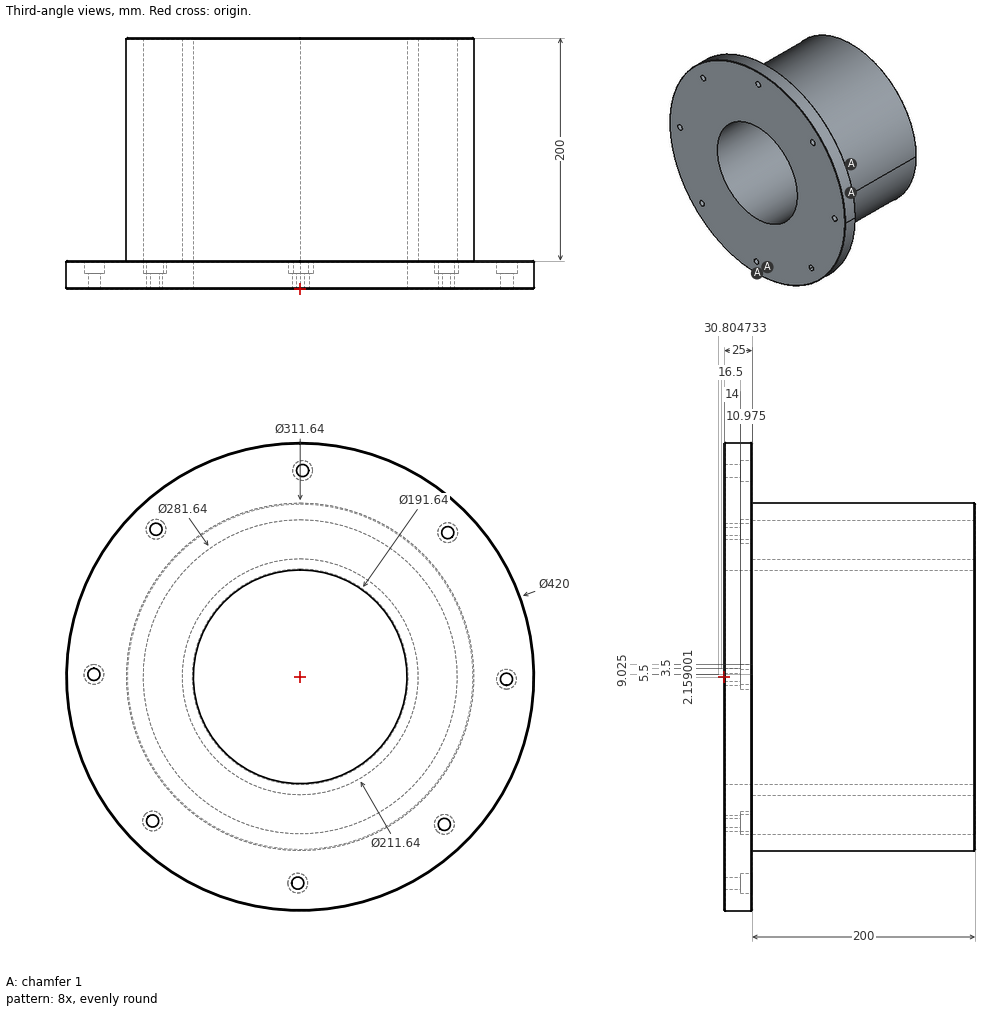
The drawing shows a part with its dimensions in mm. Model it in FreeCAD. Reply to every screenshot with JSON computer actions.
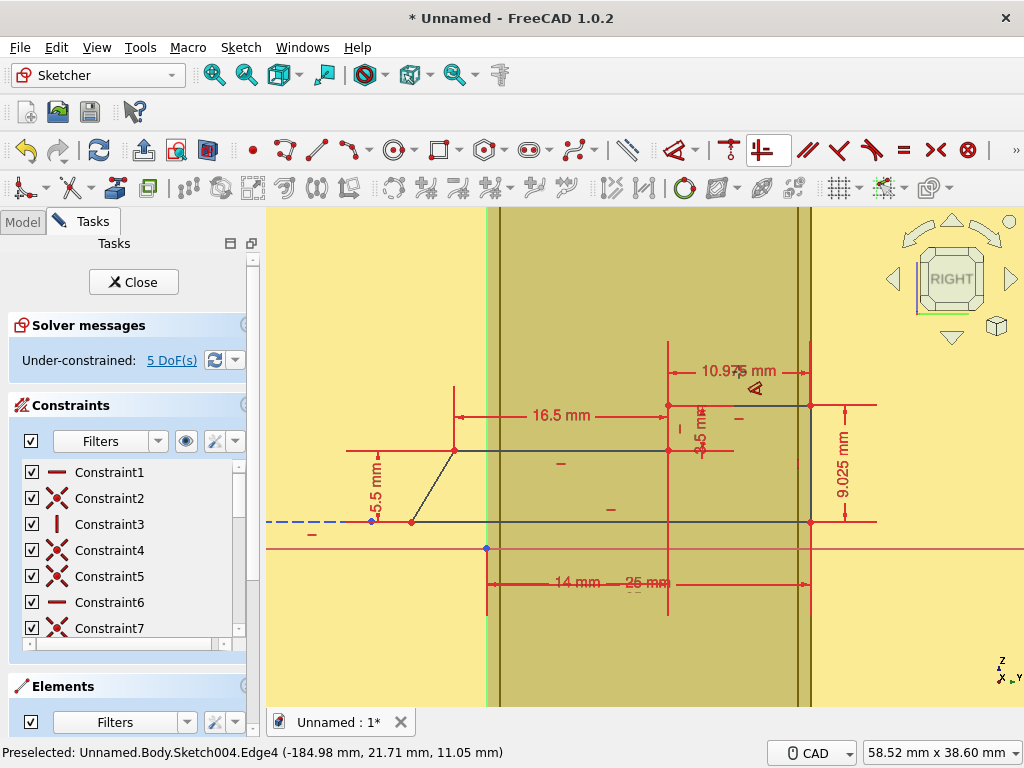
{"action": "left_click", "coordinate": [531, 522]}
{"action": "left_click", "coordinate": [611, 488]}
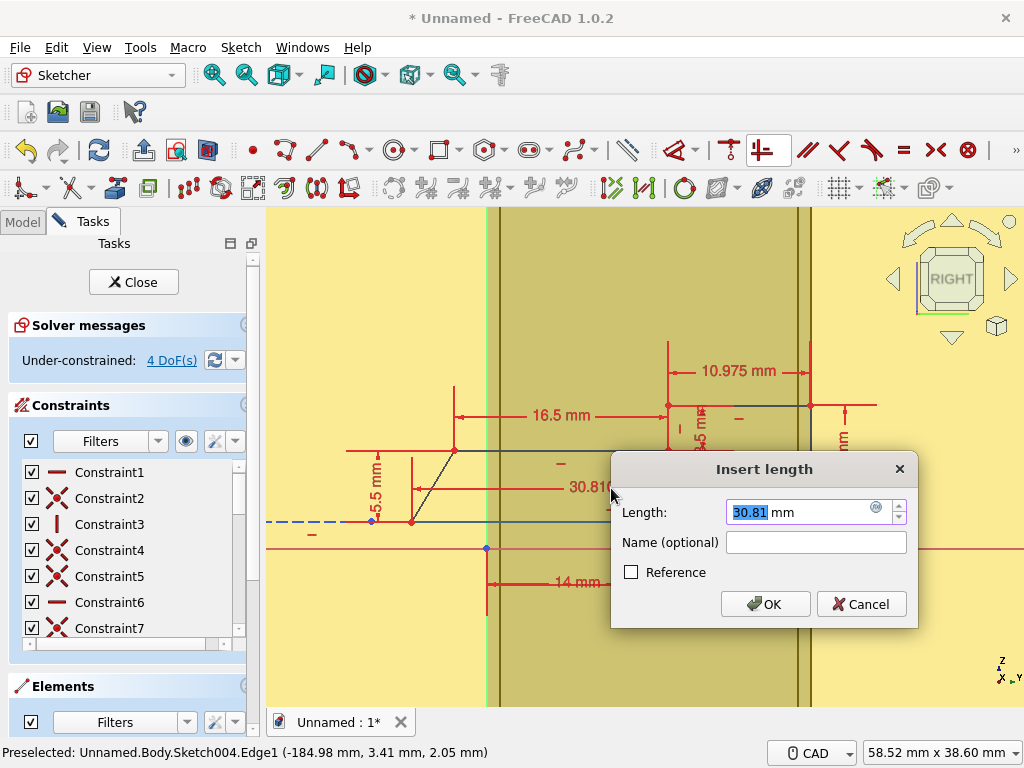
{"action": "type", "text": "30.804733"}
{"action": "key", "text": "Return"}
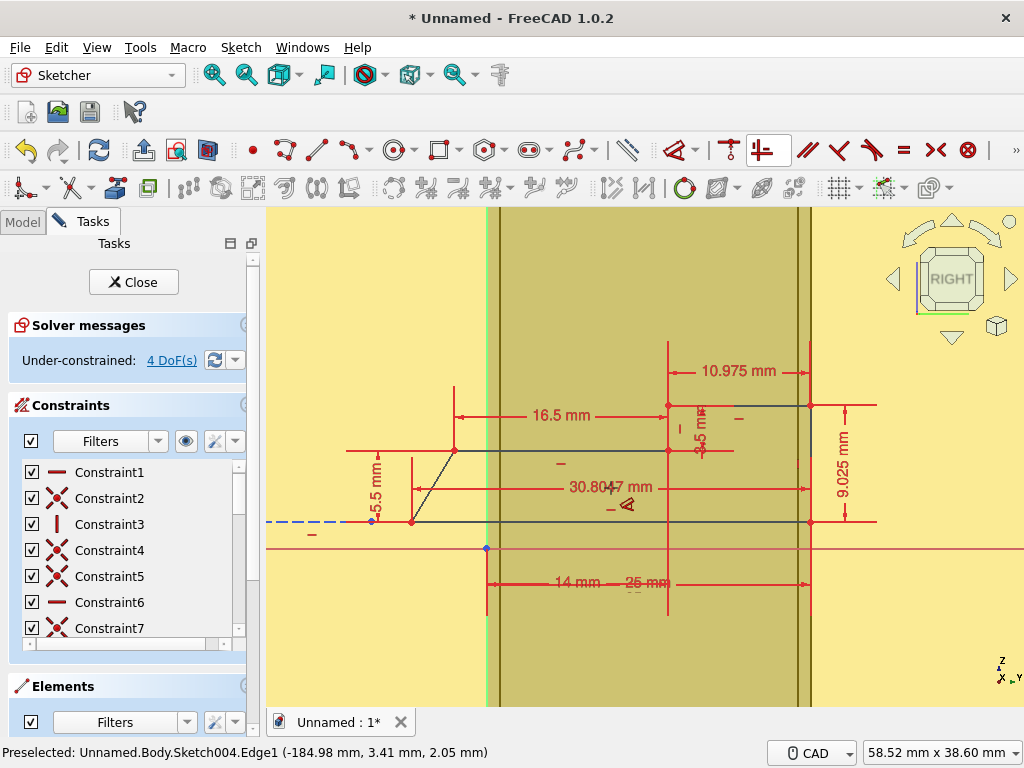
{"action": "scroll", "coordinate": [412, 522], "scroll_direction": "up", "scroll_amount": 2}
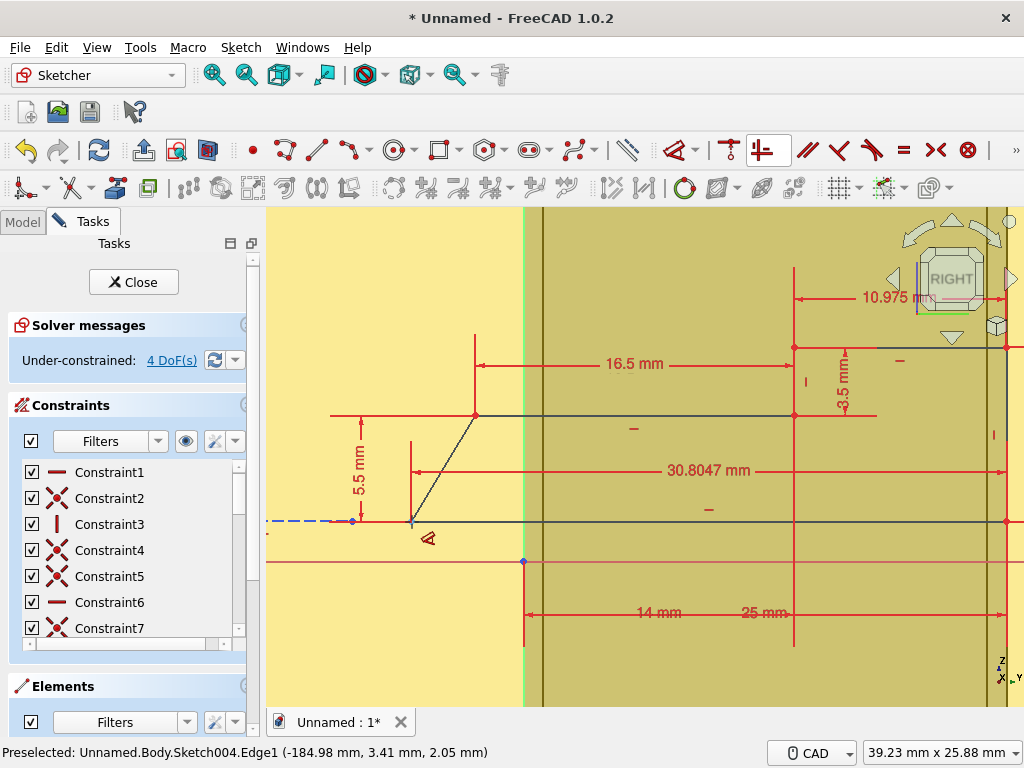
{"action": "left_click", "coordinate": [411, 522]}
{"action": "left_click", "coordinate": [377, 542]}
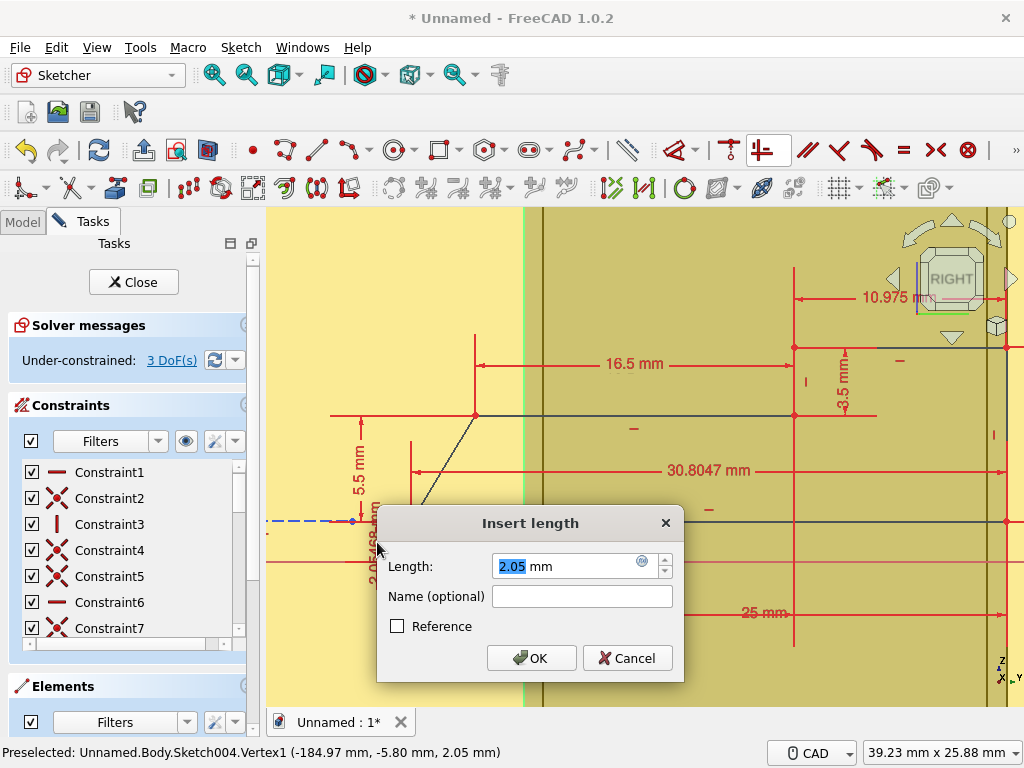
{"action": "type", "text": "2.159001"}
{"action": "key", "text": "Return"}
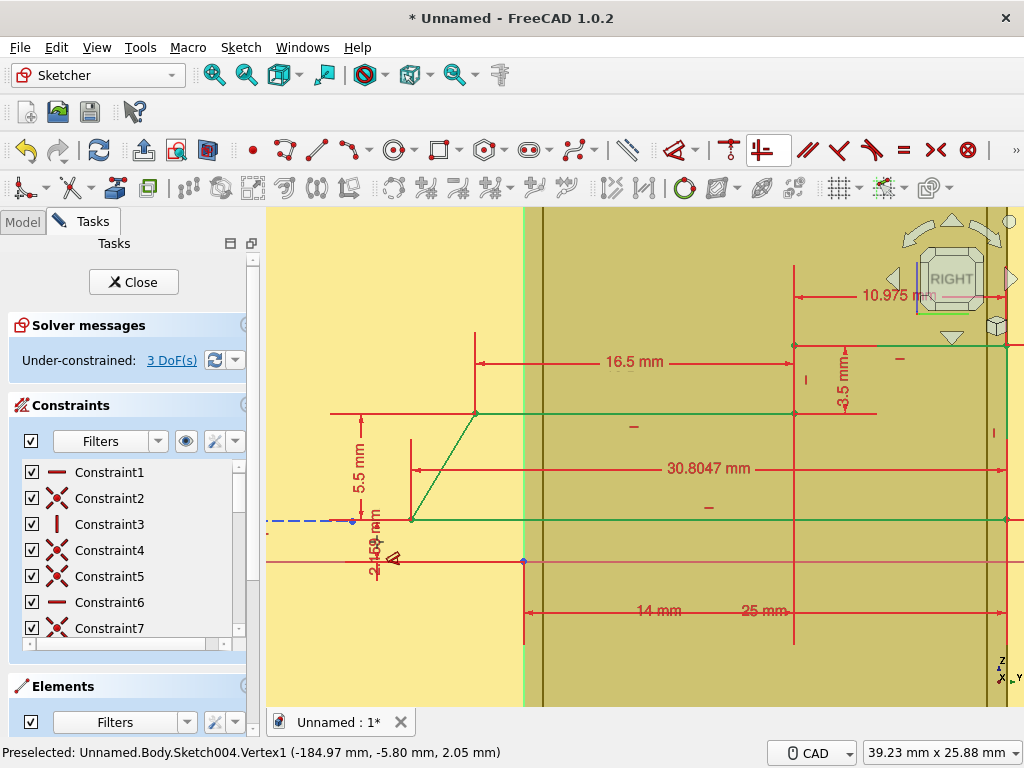
{"action": "left_click", "coordinate": [352, 521]}
{"action": "left_click", "coordinate": [558, 541]}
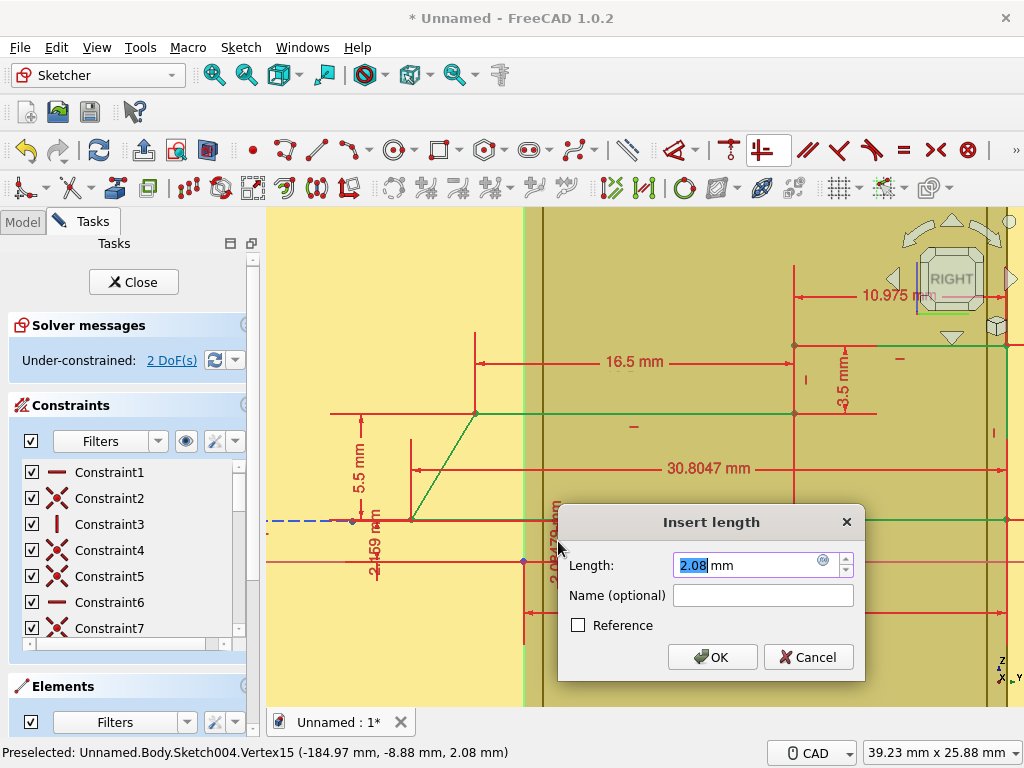
{"action": "type", "text": "2.159001"}
{"action": "key", "text": "Return"}
{"action": "key", "text": "Escape"}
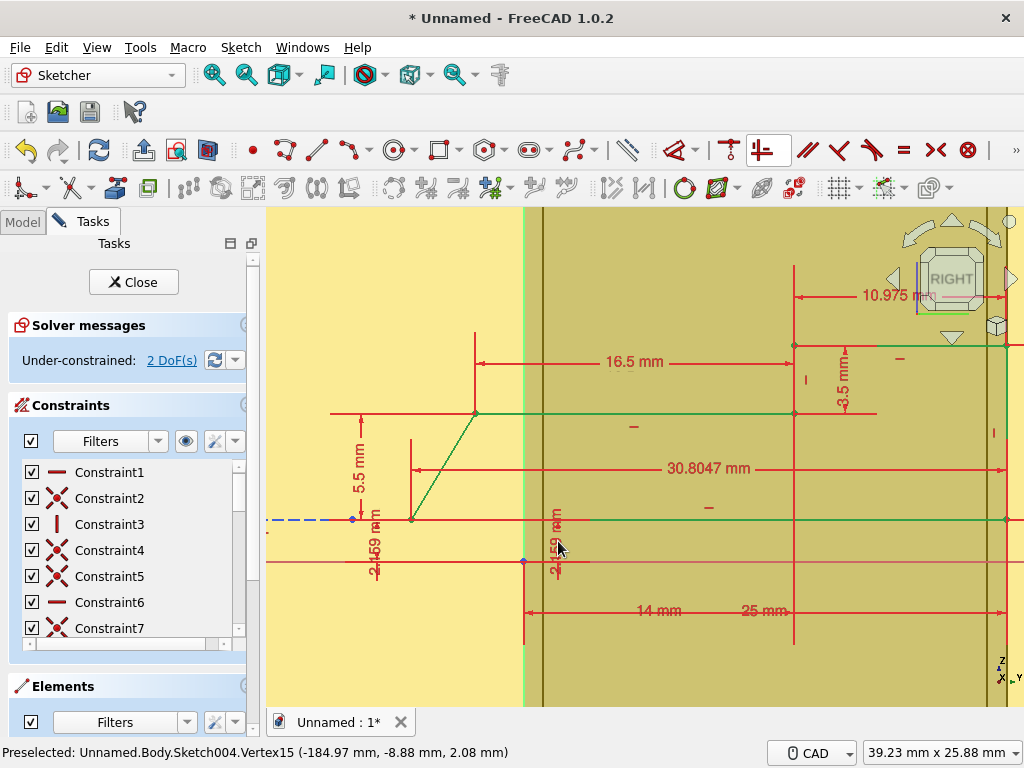
{"action": "left_click", "coordinate": [134, 282]}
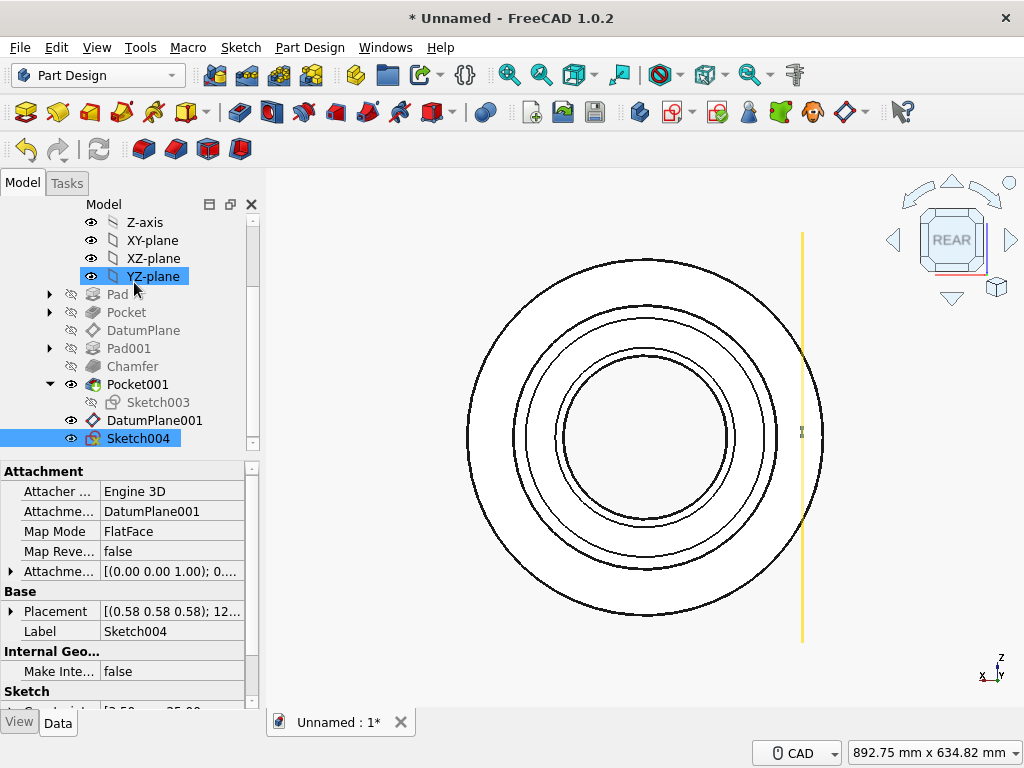
{"action": "left_click", "coordinate": [304, 112]}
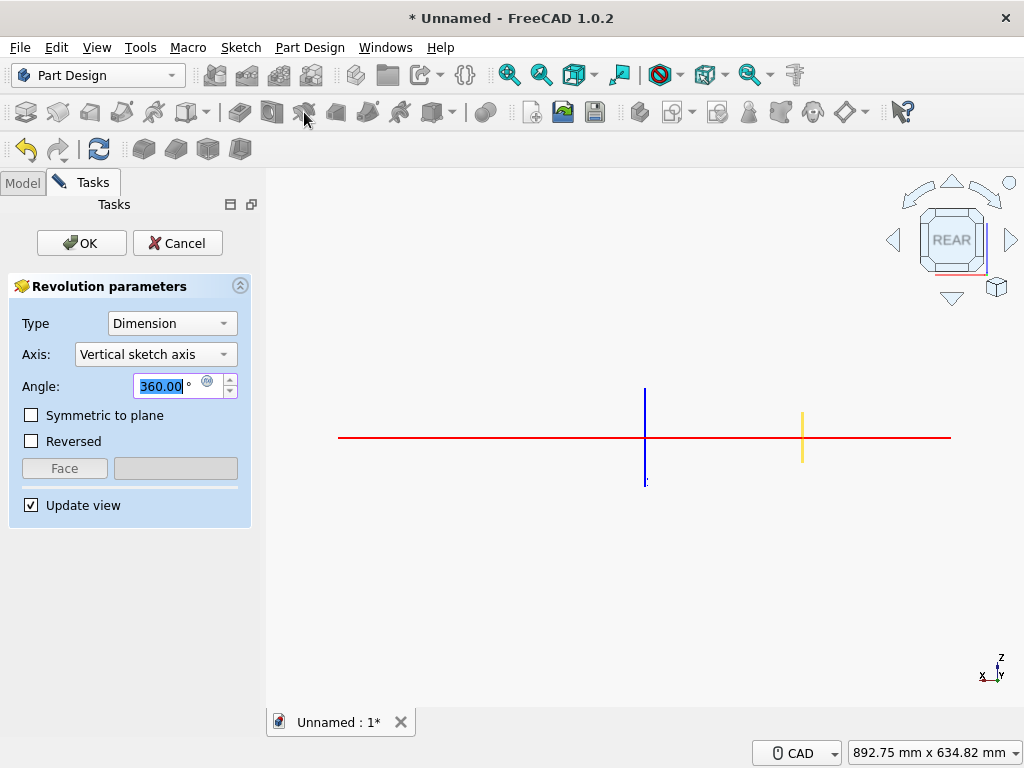
{"action": "left_click", "coordinate": [156, 354]}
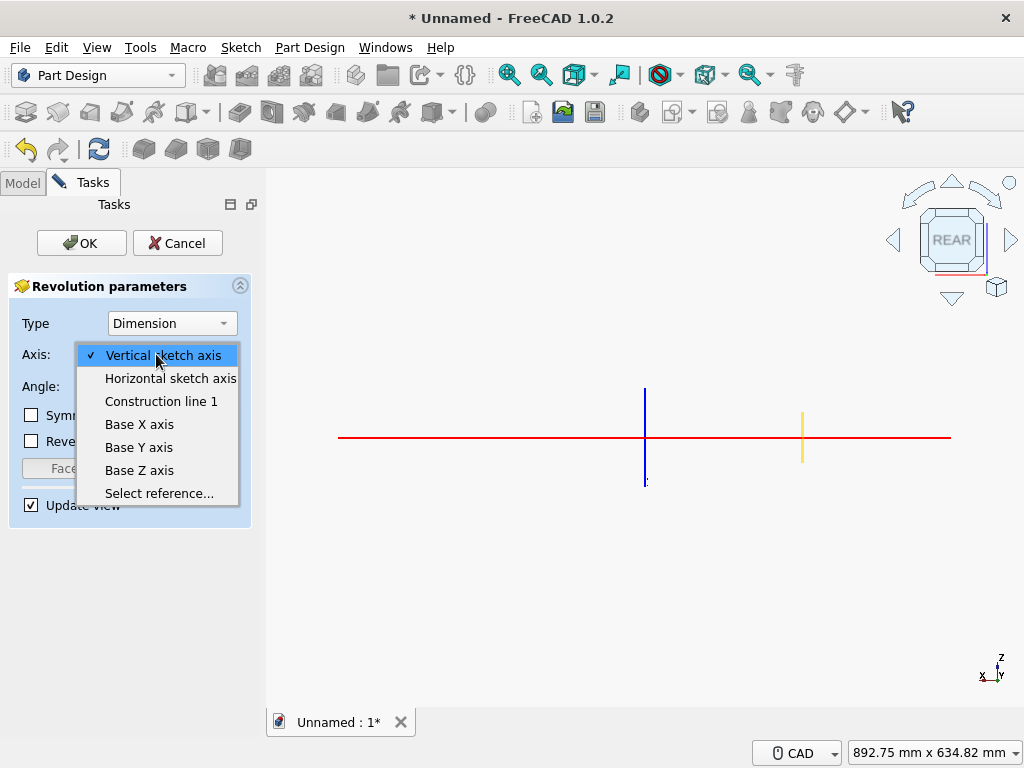
{"action": "left_click", "coordinate": [156, 402]}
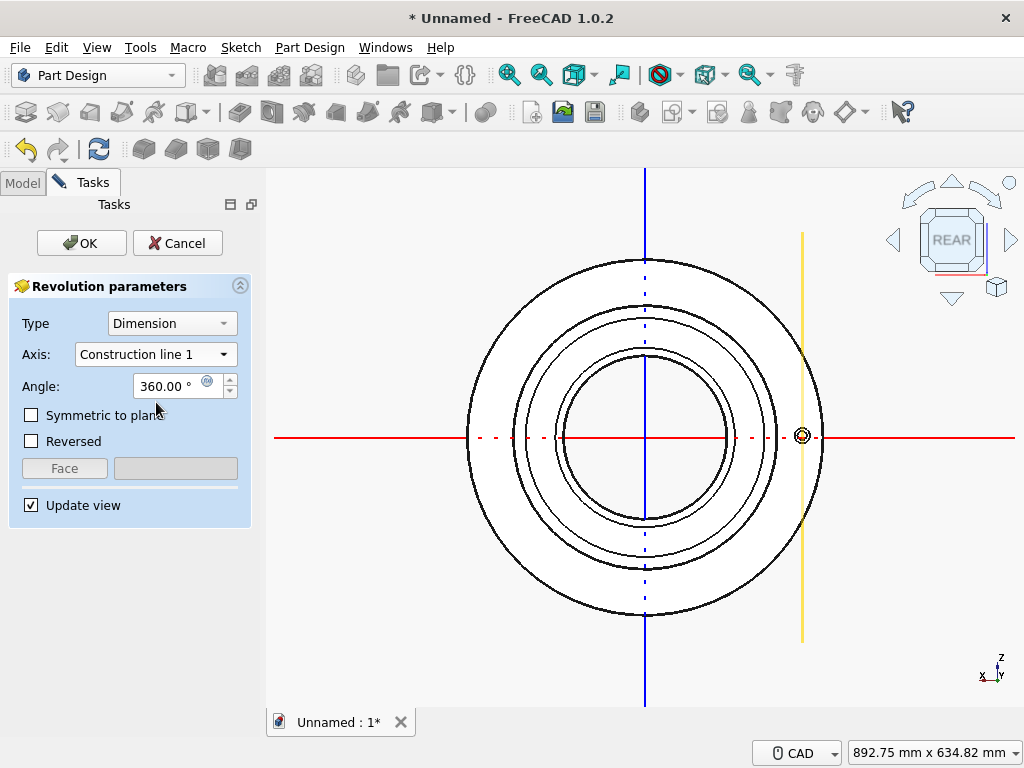
{"action": "left_click", "coordinate": [82, 243]}